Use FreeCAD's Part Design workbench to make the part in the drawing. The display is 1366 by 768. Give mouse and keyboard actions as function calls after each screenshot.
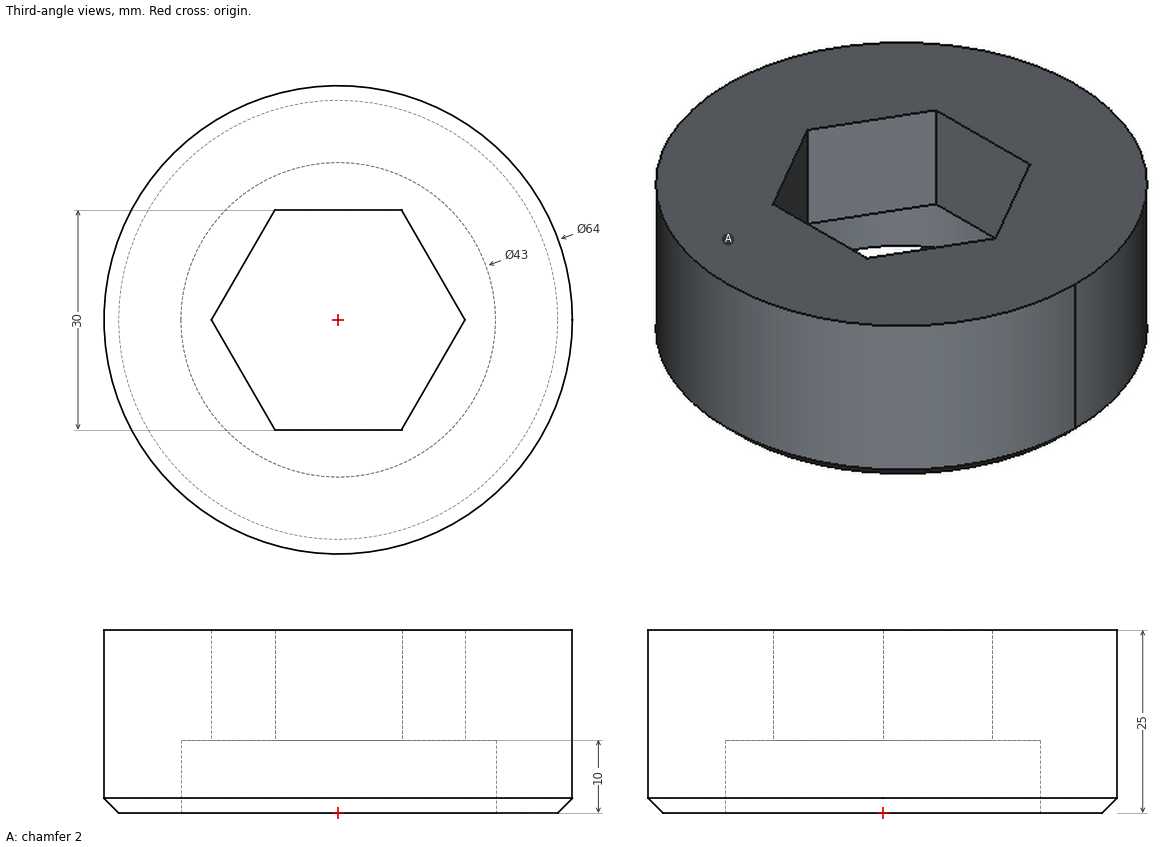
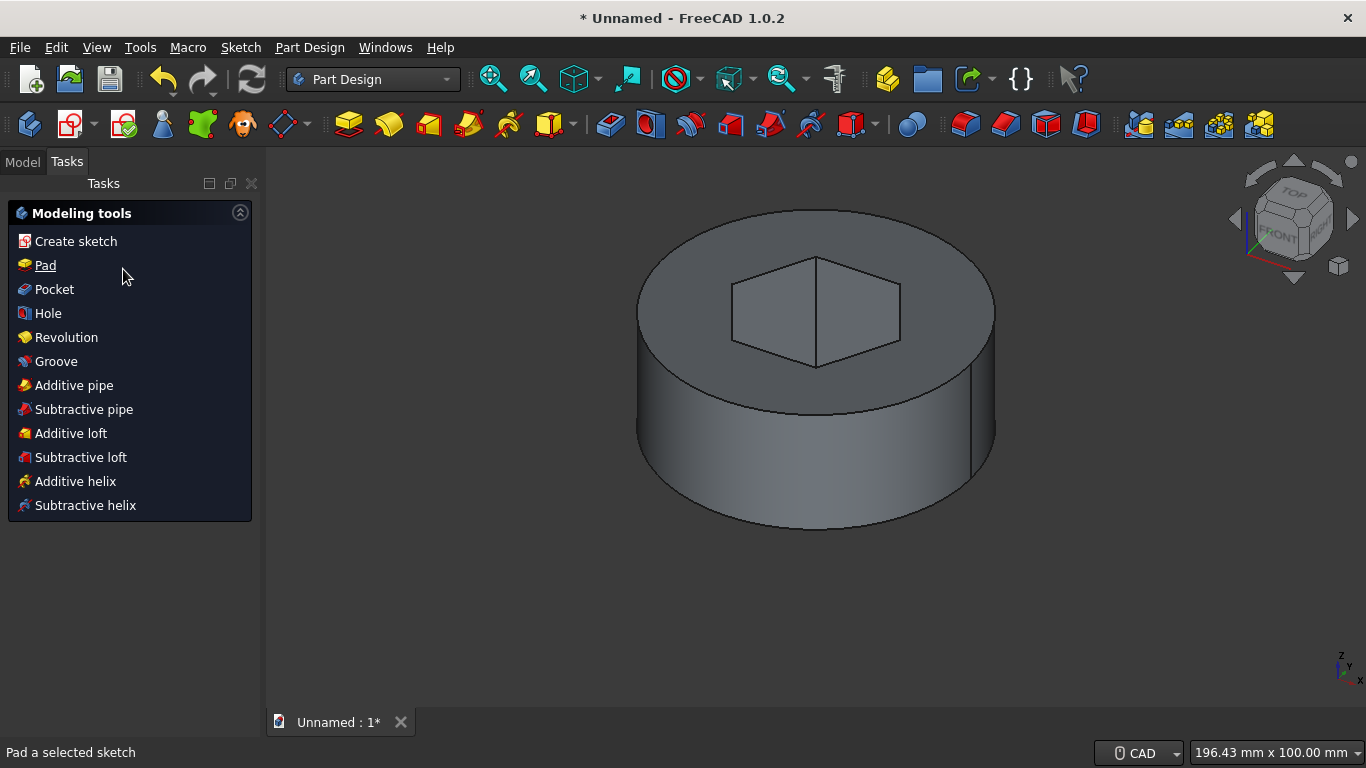
click(612, 124)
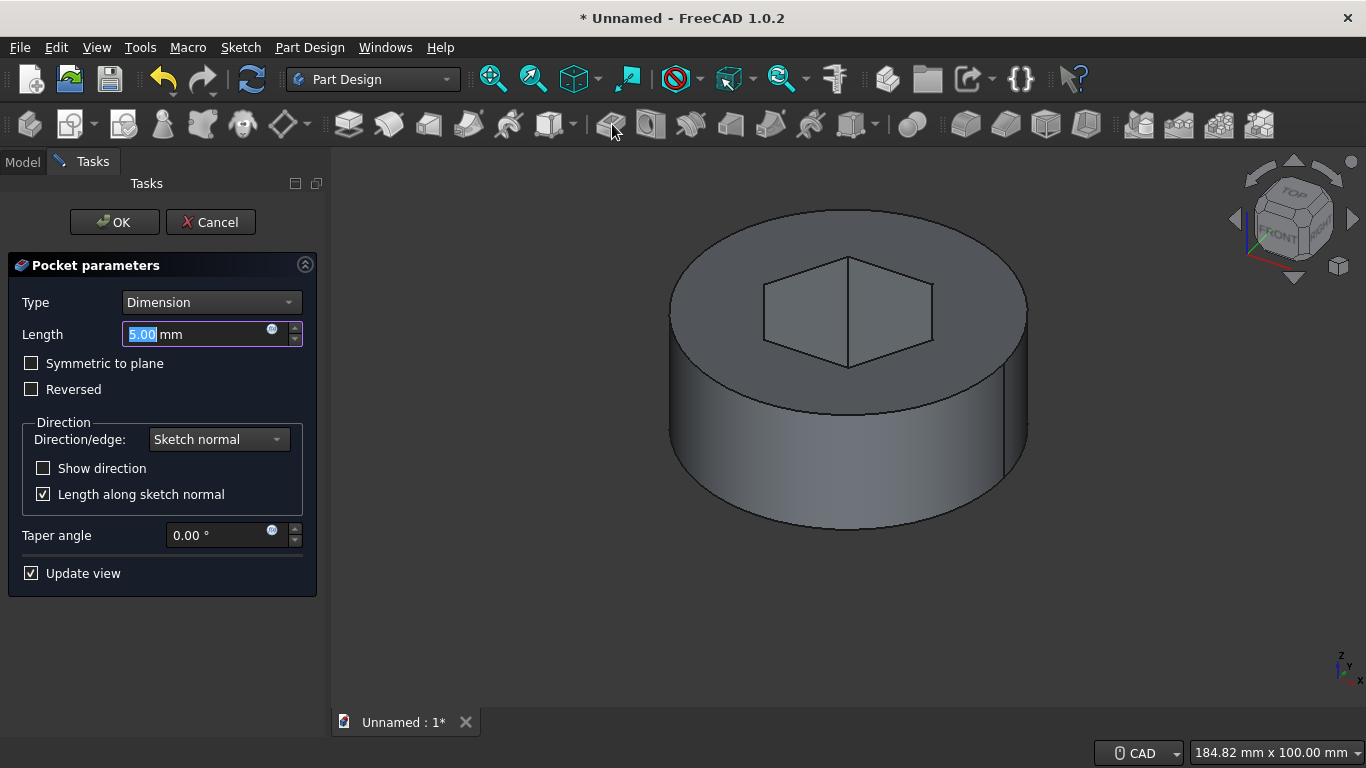
text(10)
key(Tab)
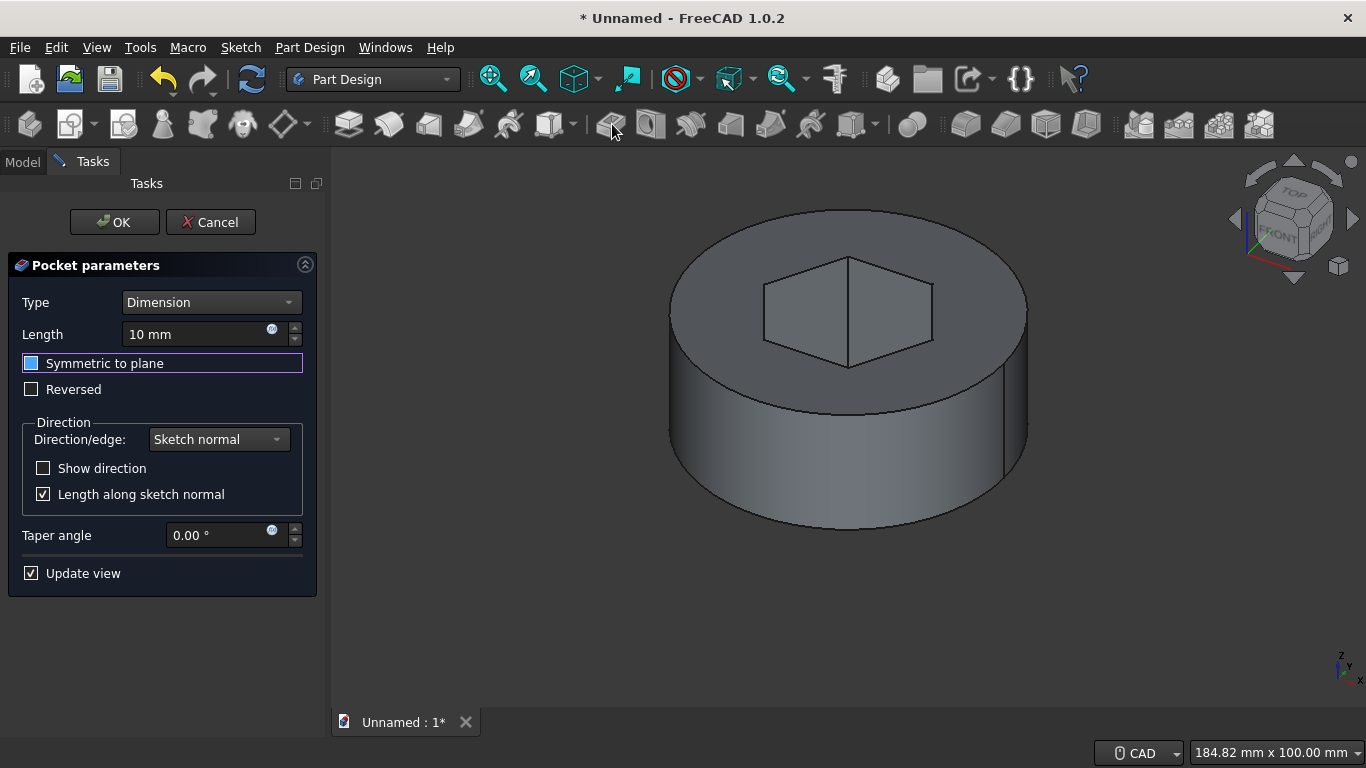
click(30, 389)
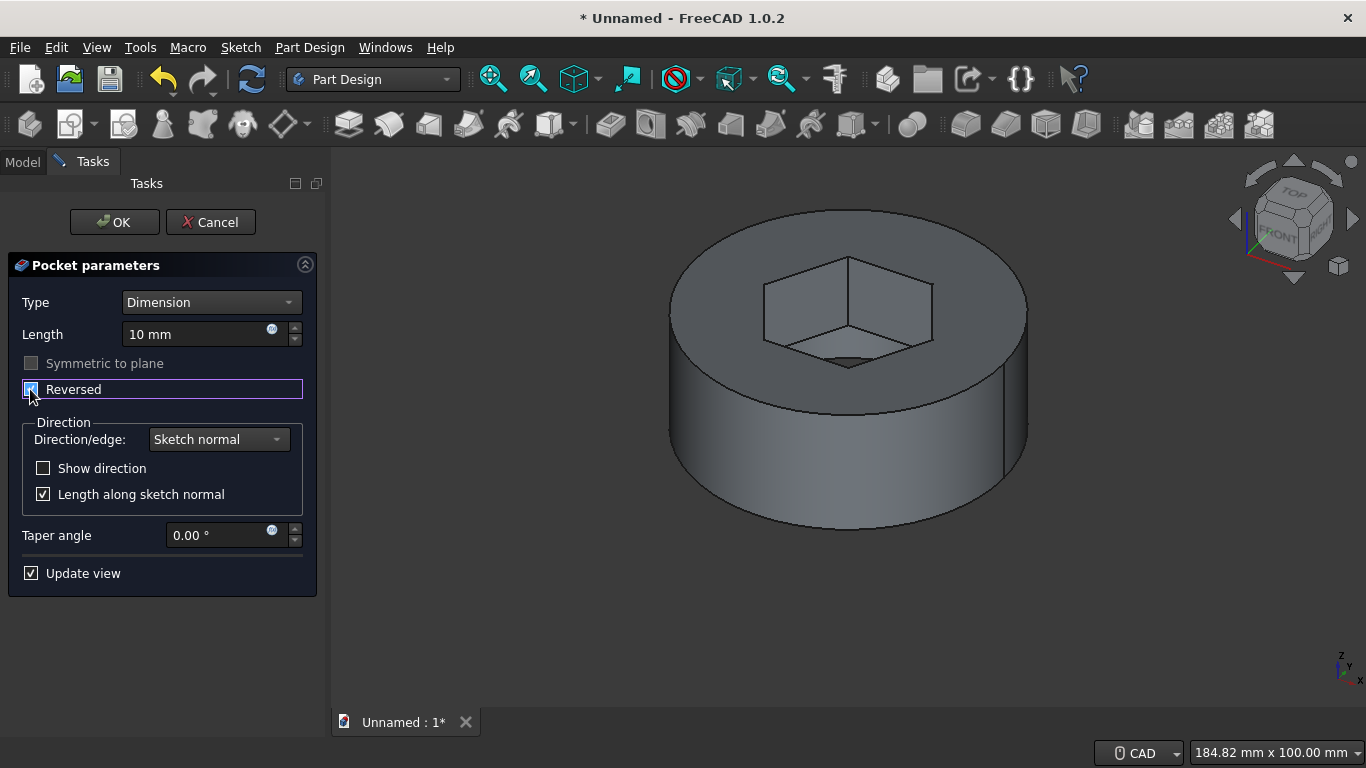
click(115, 222)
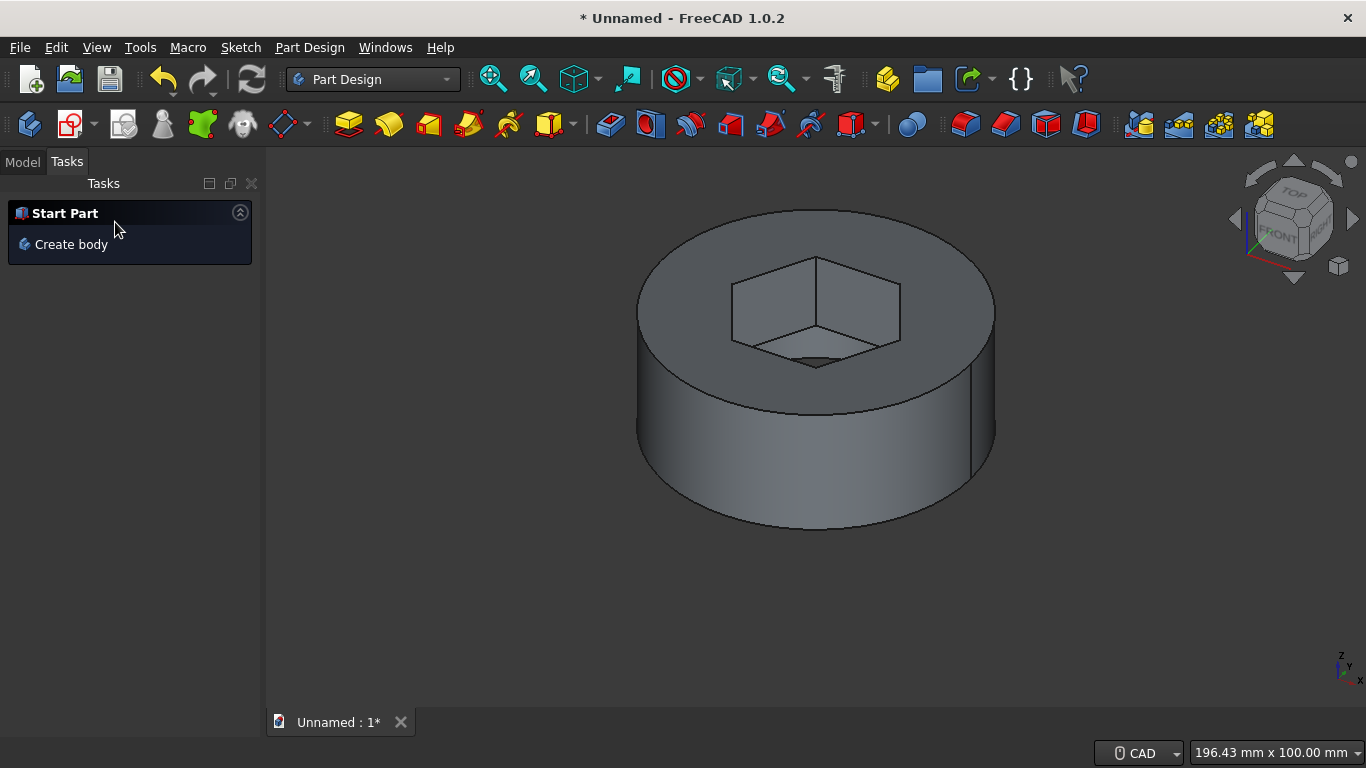
click(779, 527)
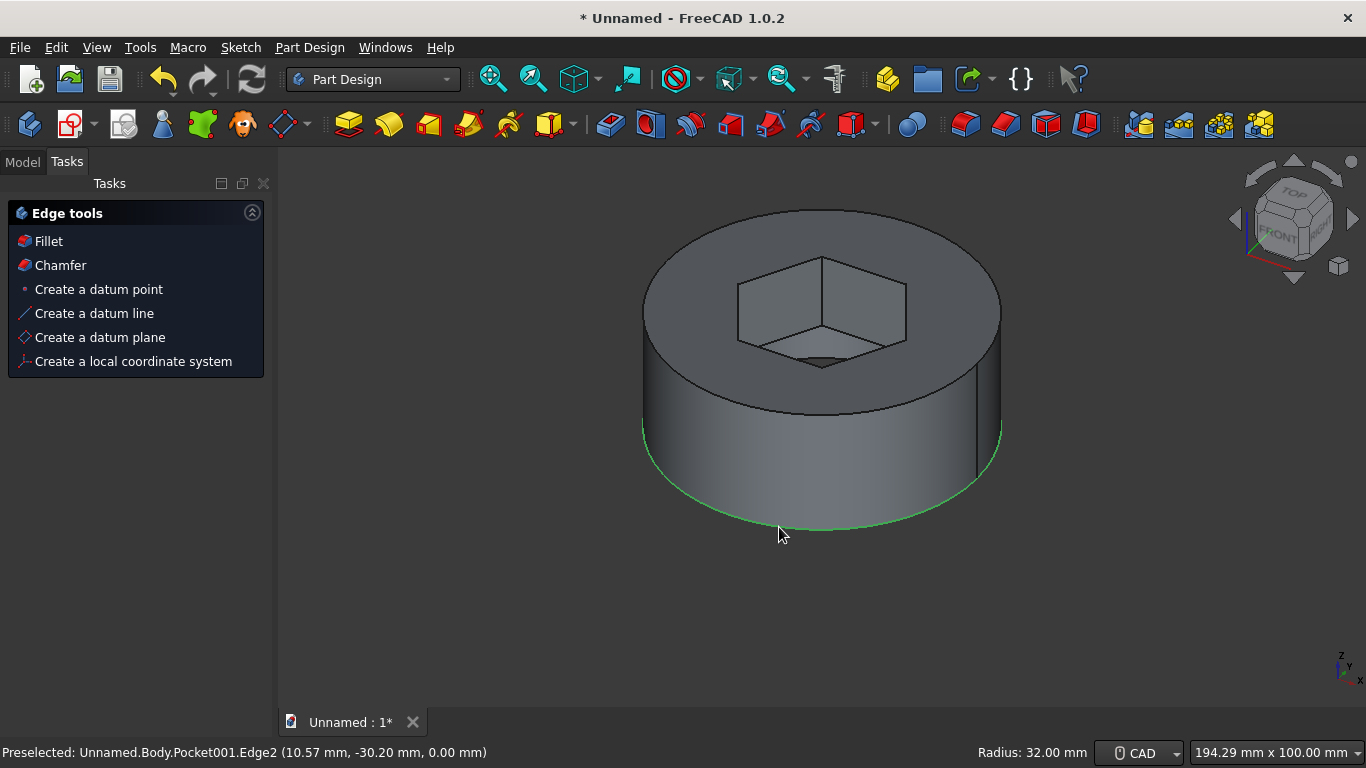
click(1006, 124)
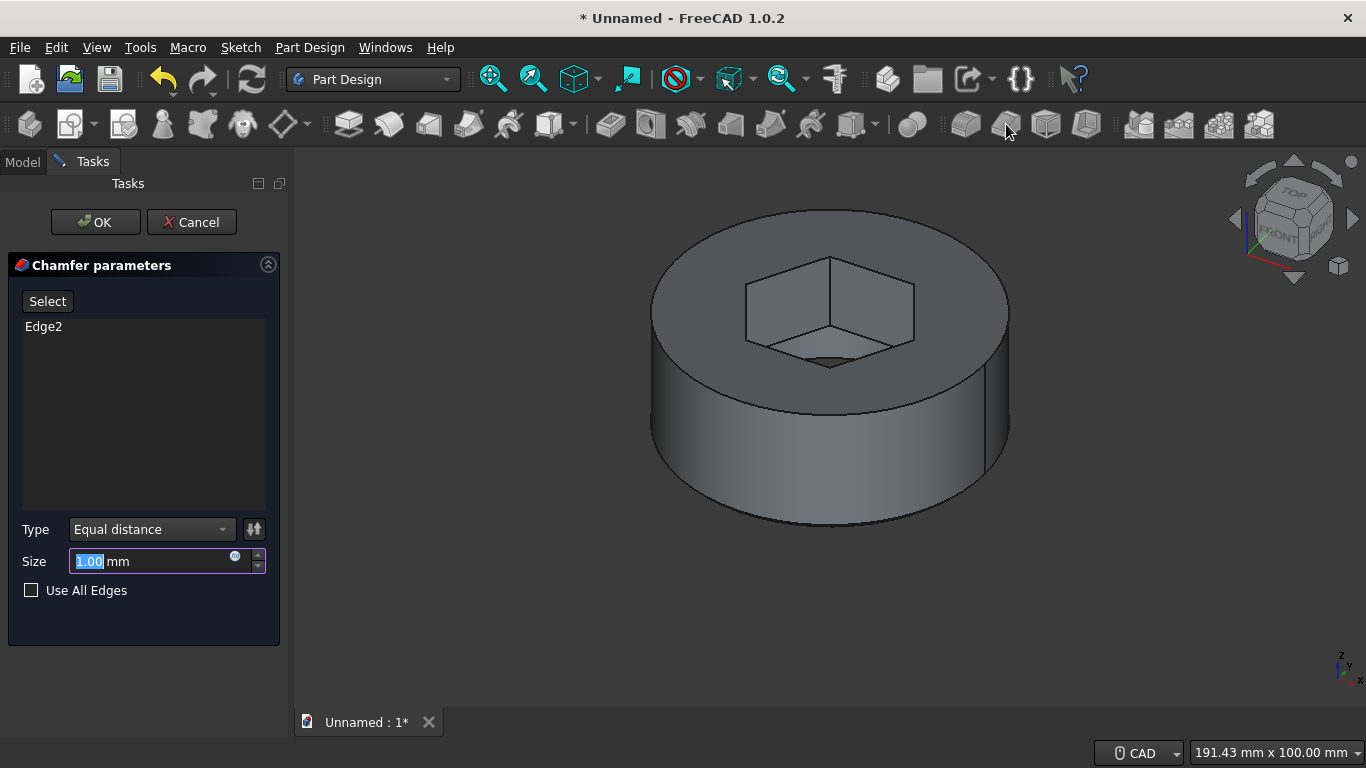
text(2)
key(Tab)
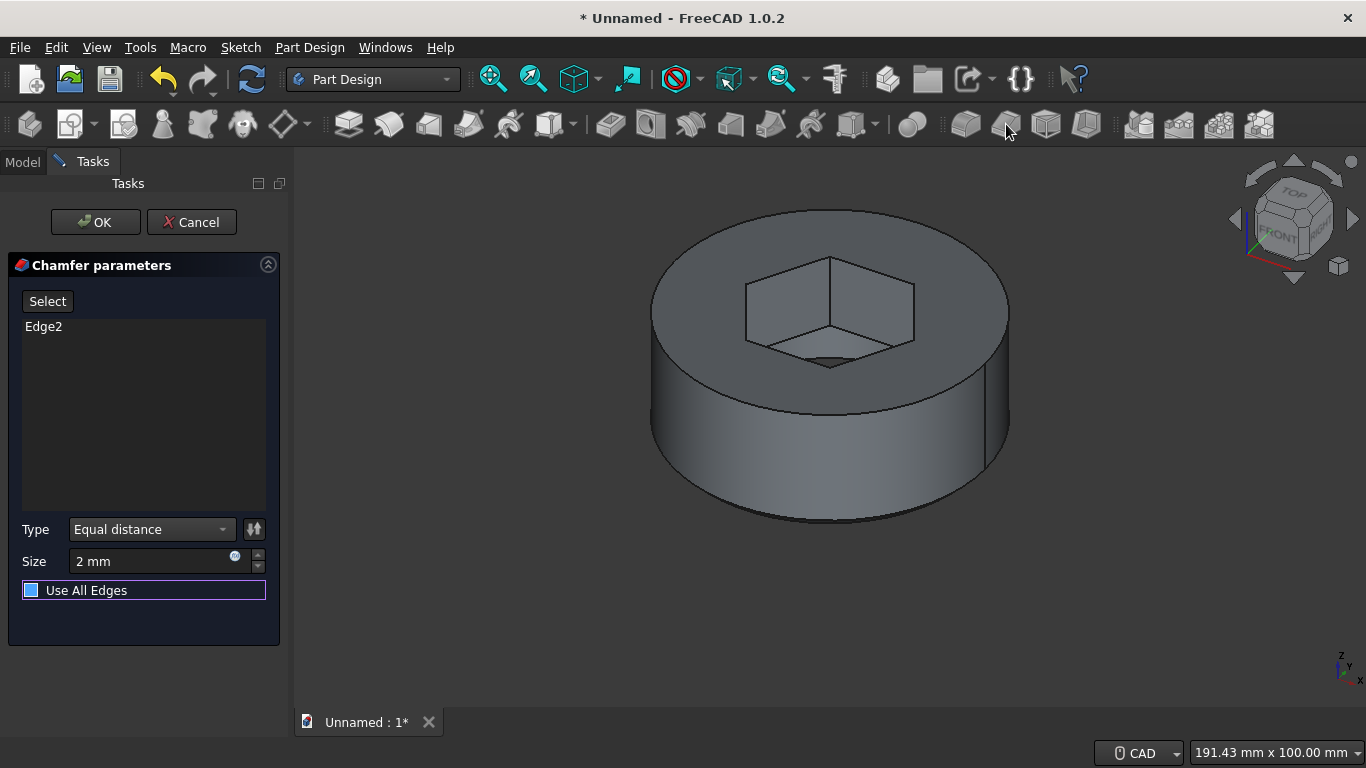
click(96, 222)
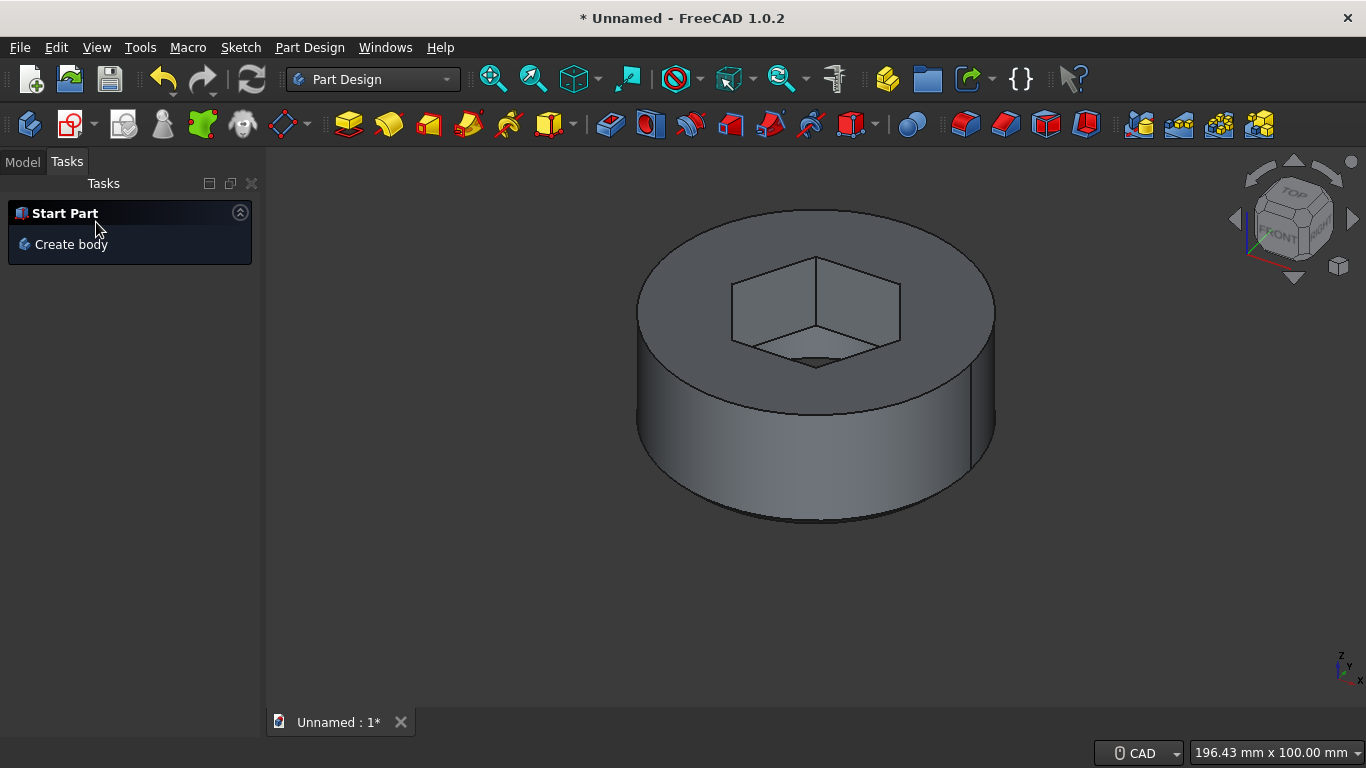
key(0)